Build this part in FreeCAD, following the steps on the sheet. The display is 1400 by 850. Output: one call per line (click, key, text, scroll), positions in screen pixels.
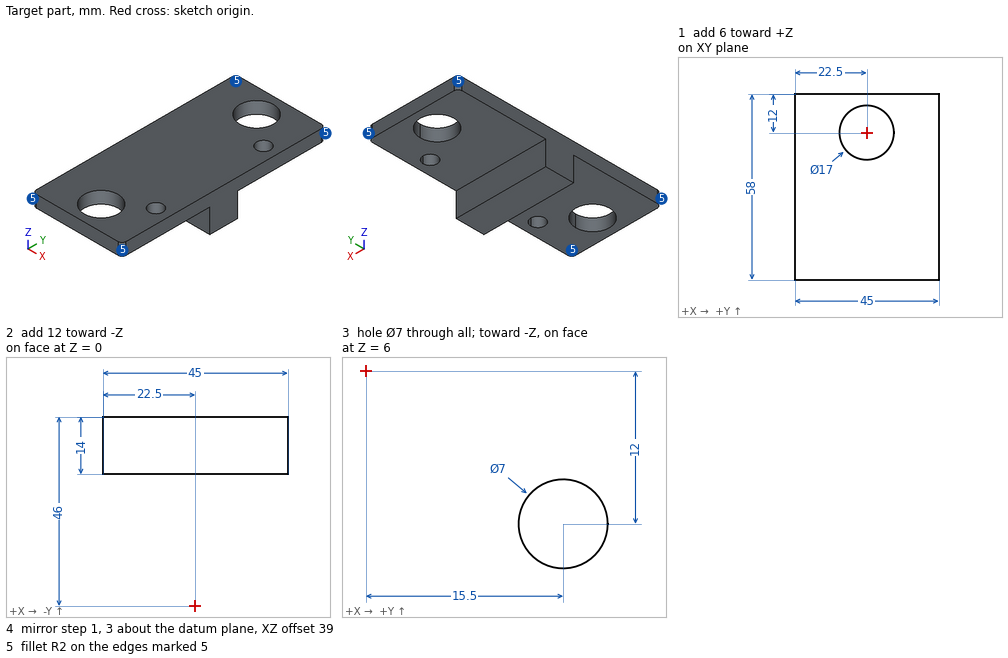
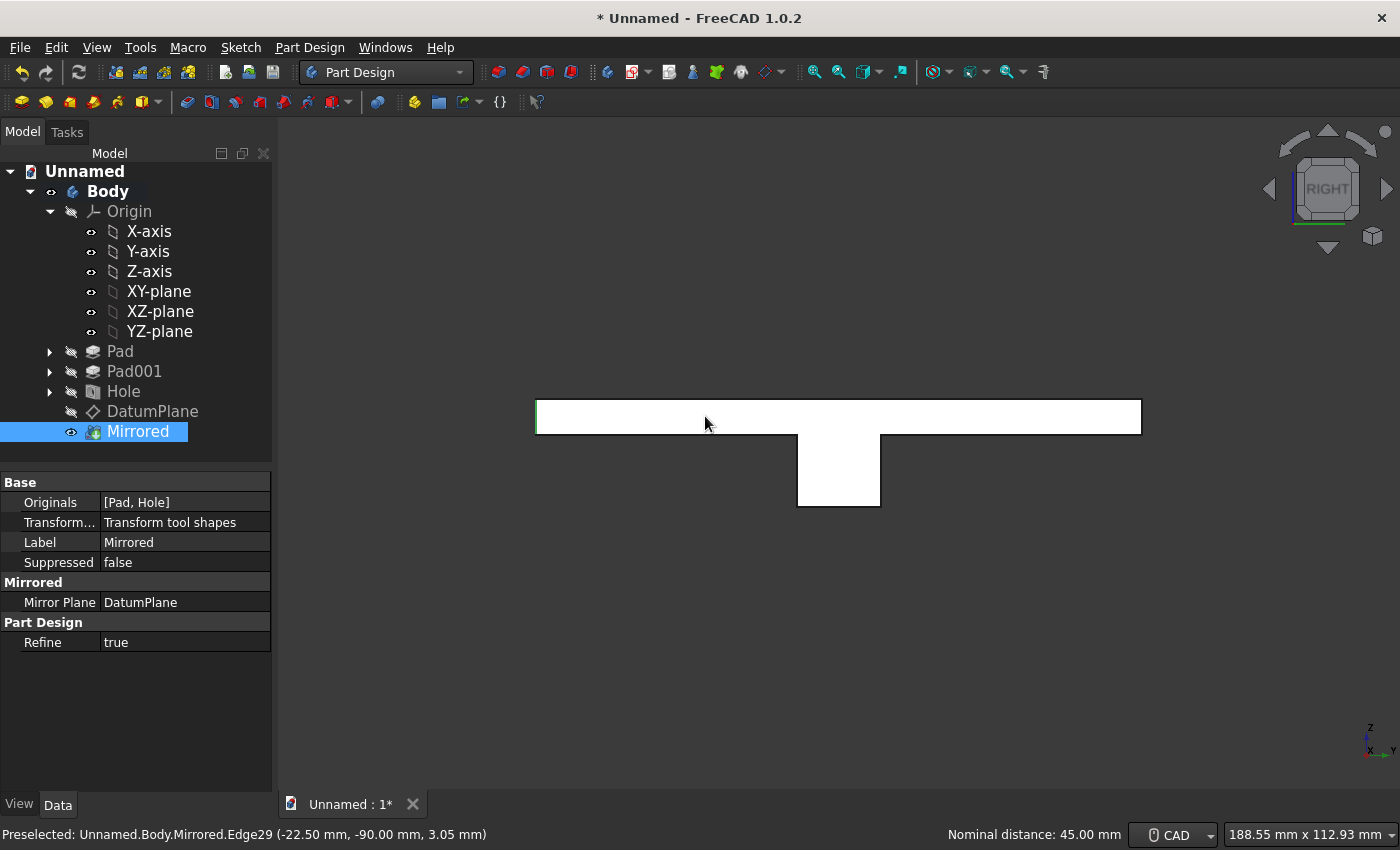
click(1142, 416, ctrl)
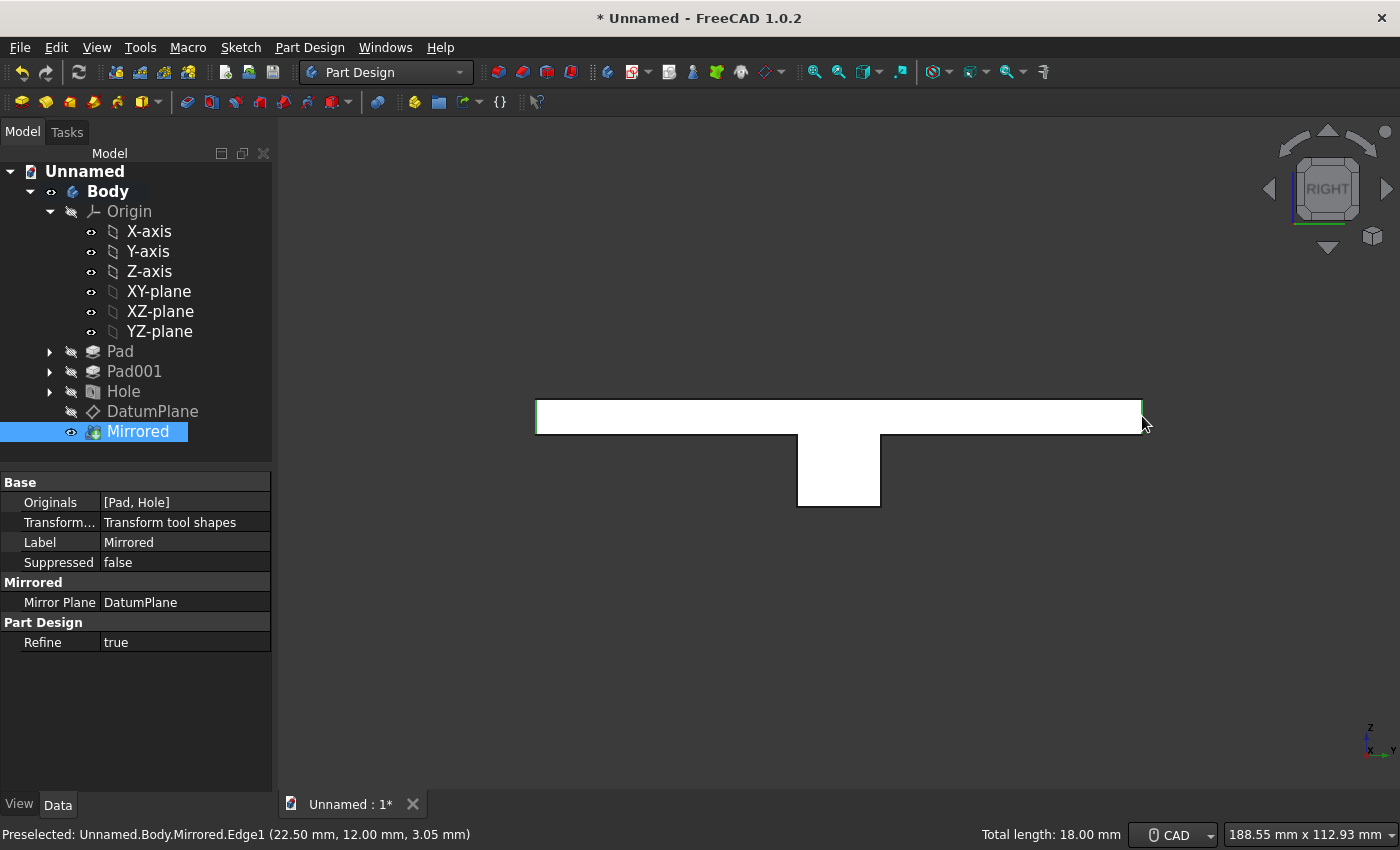
key(5)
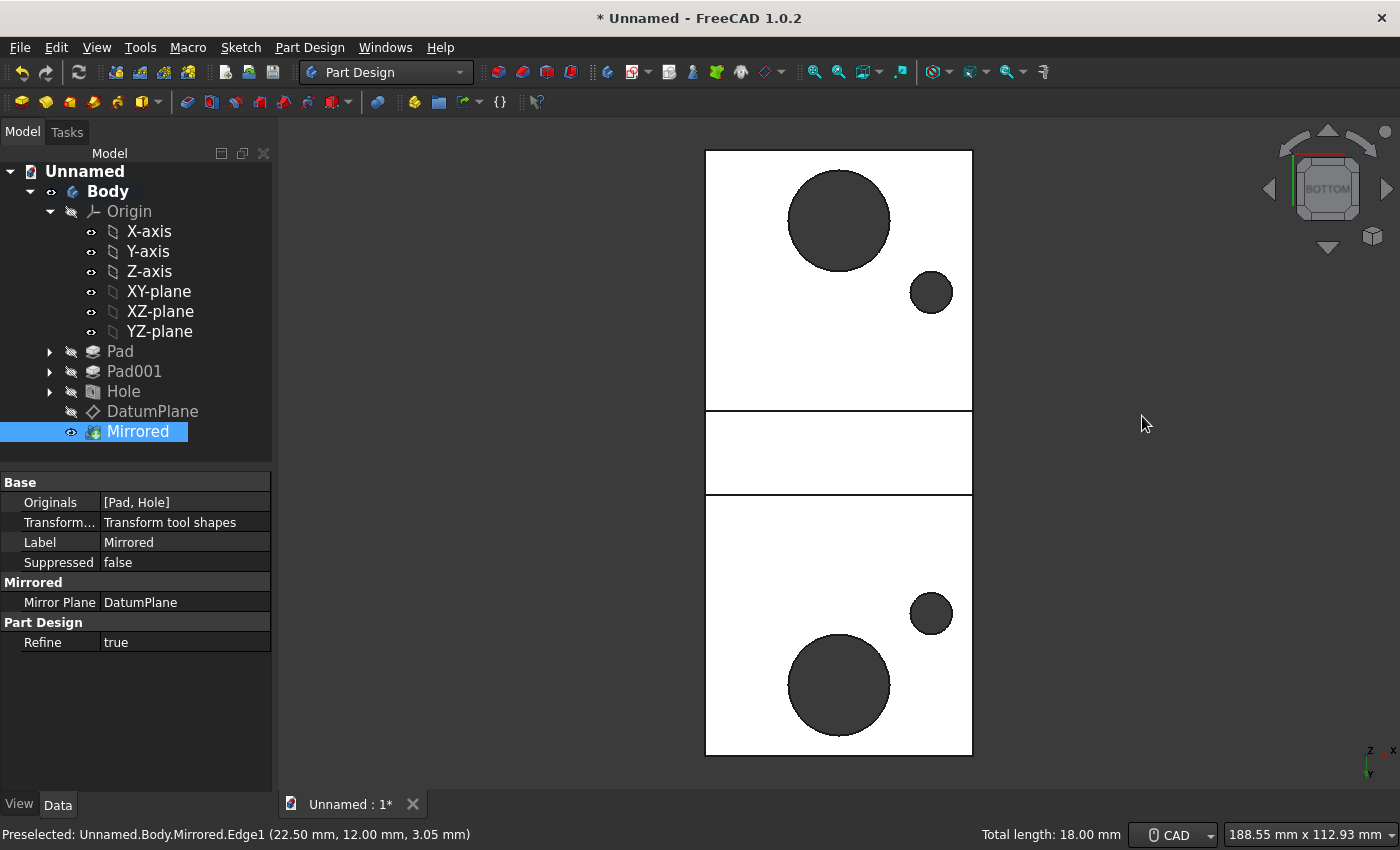
key(4)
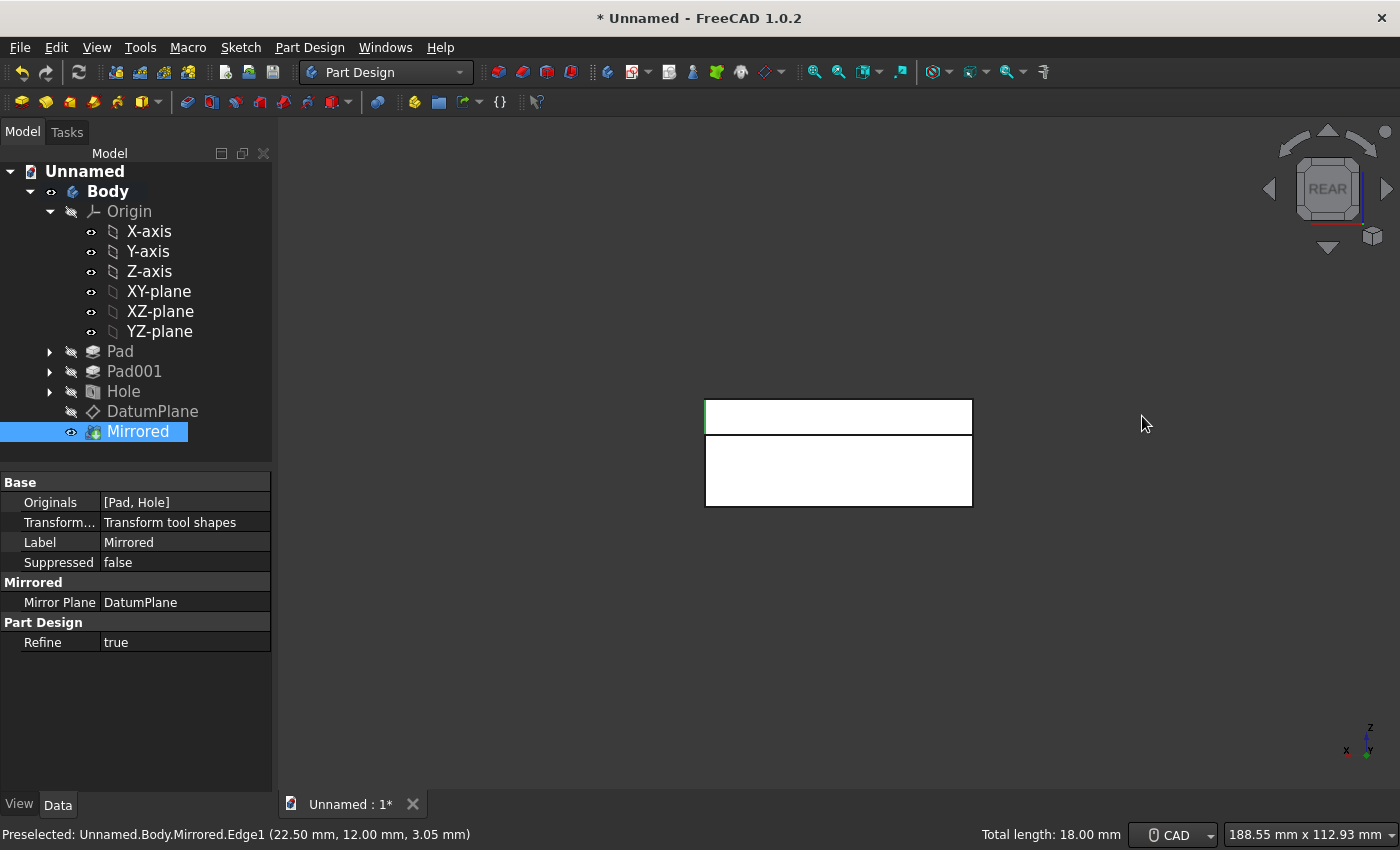
click(816, 72)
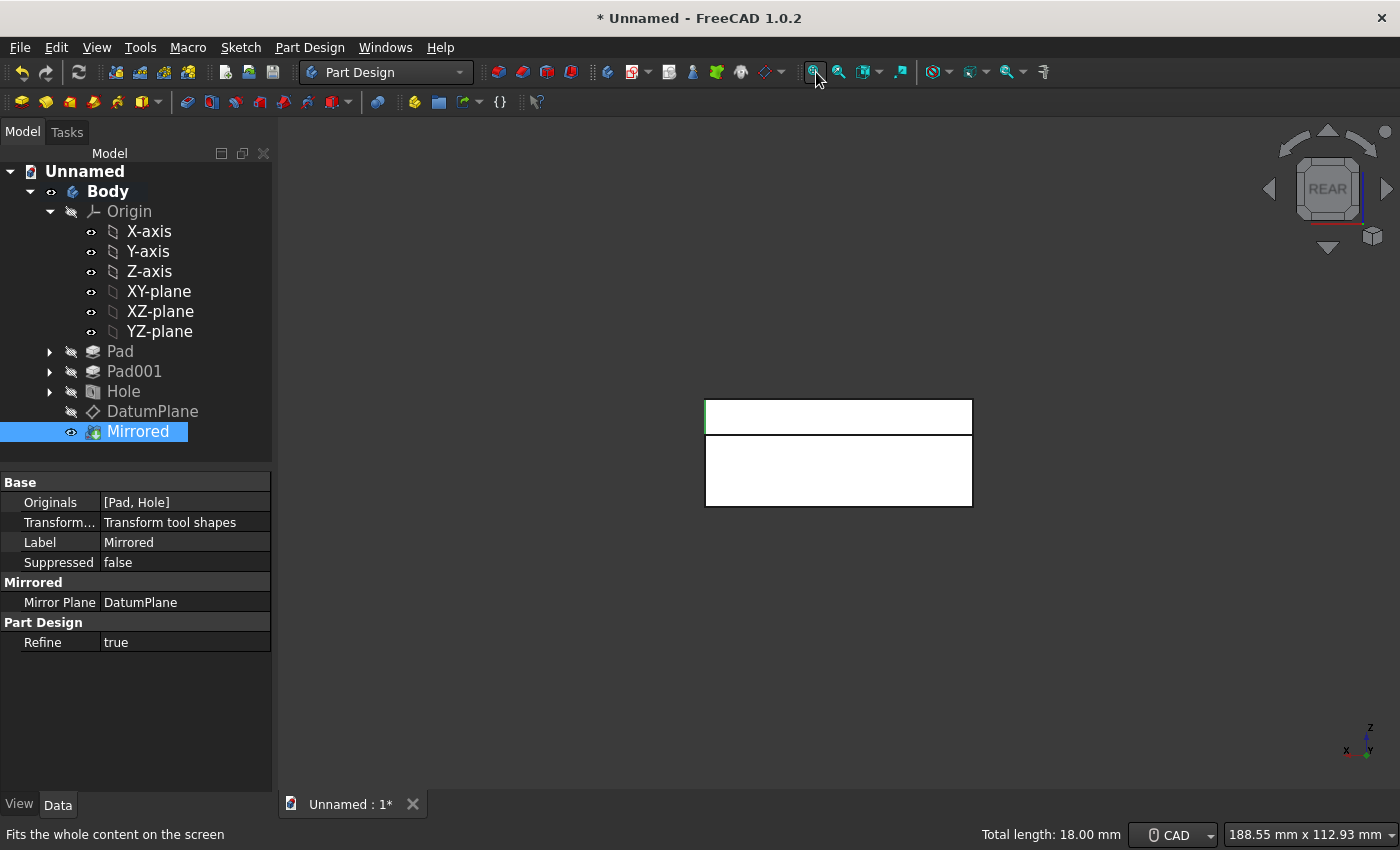
click(973, 416, ctrl)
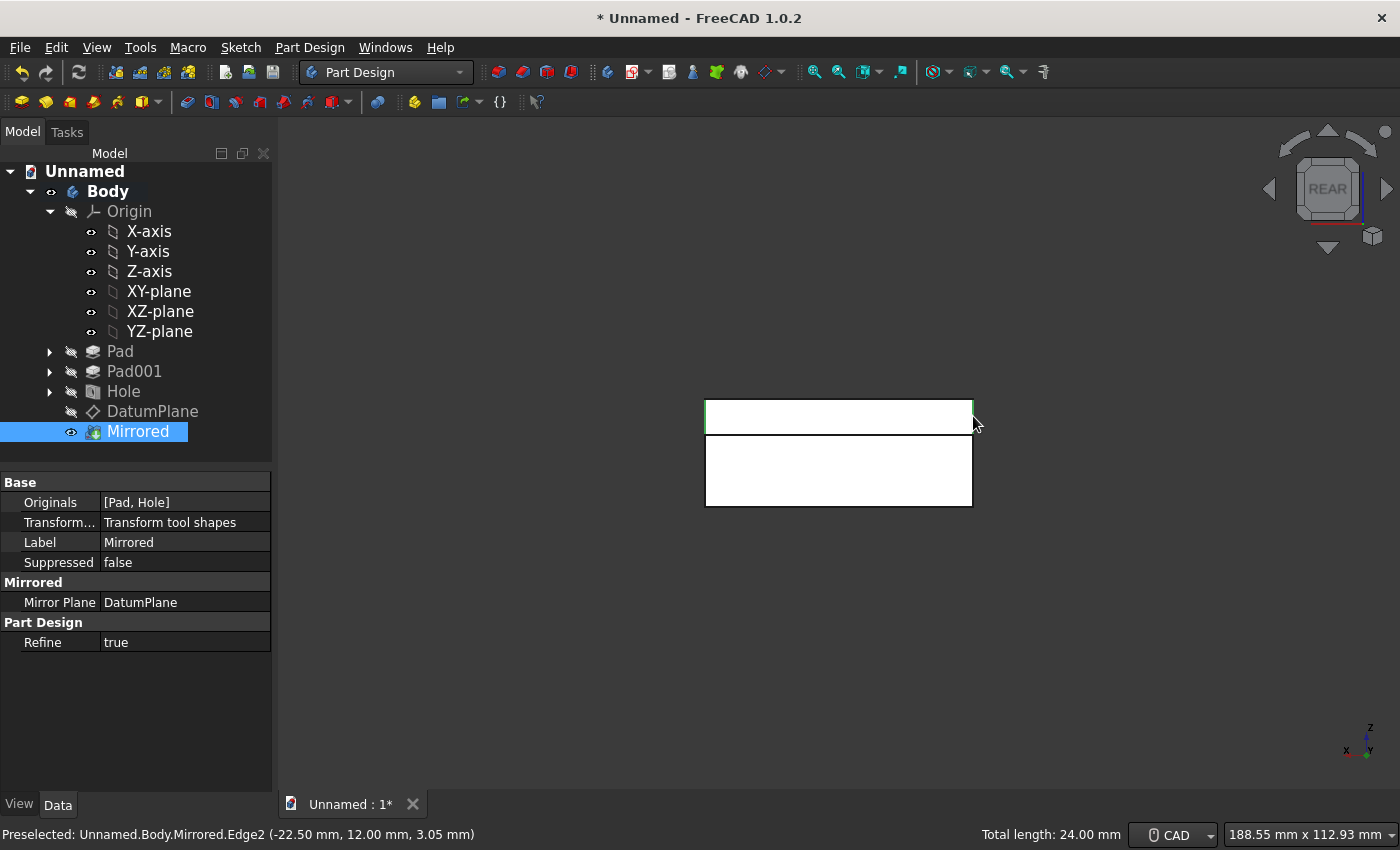
click(500, 72)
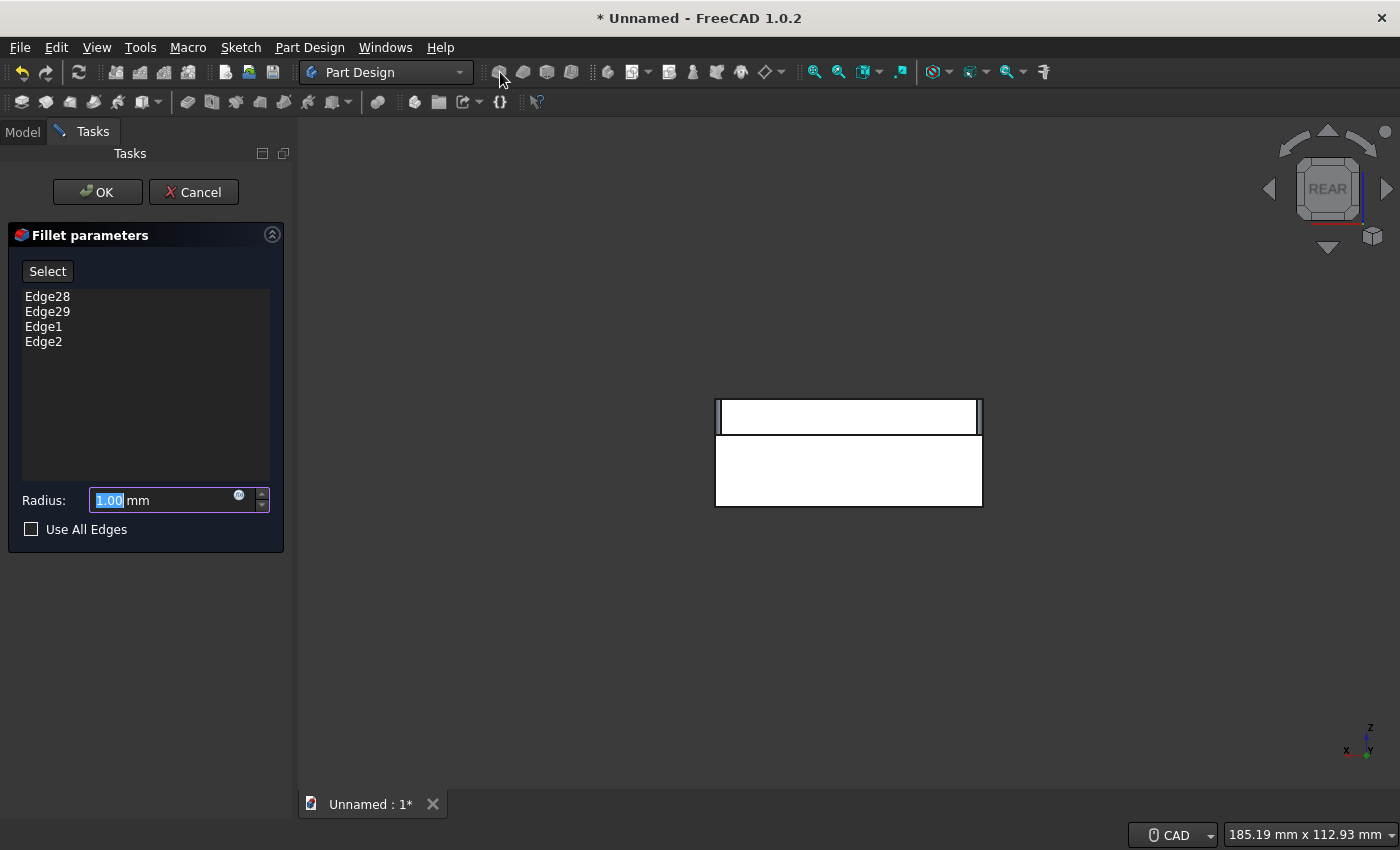
text(2)
key(Tab)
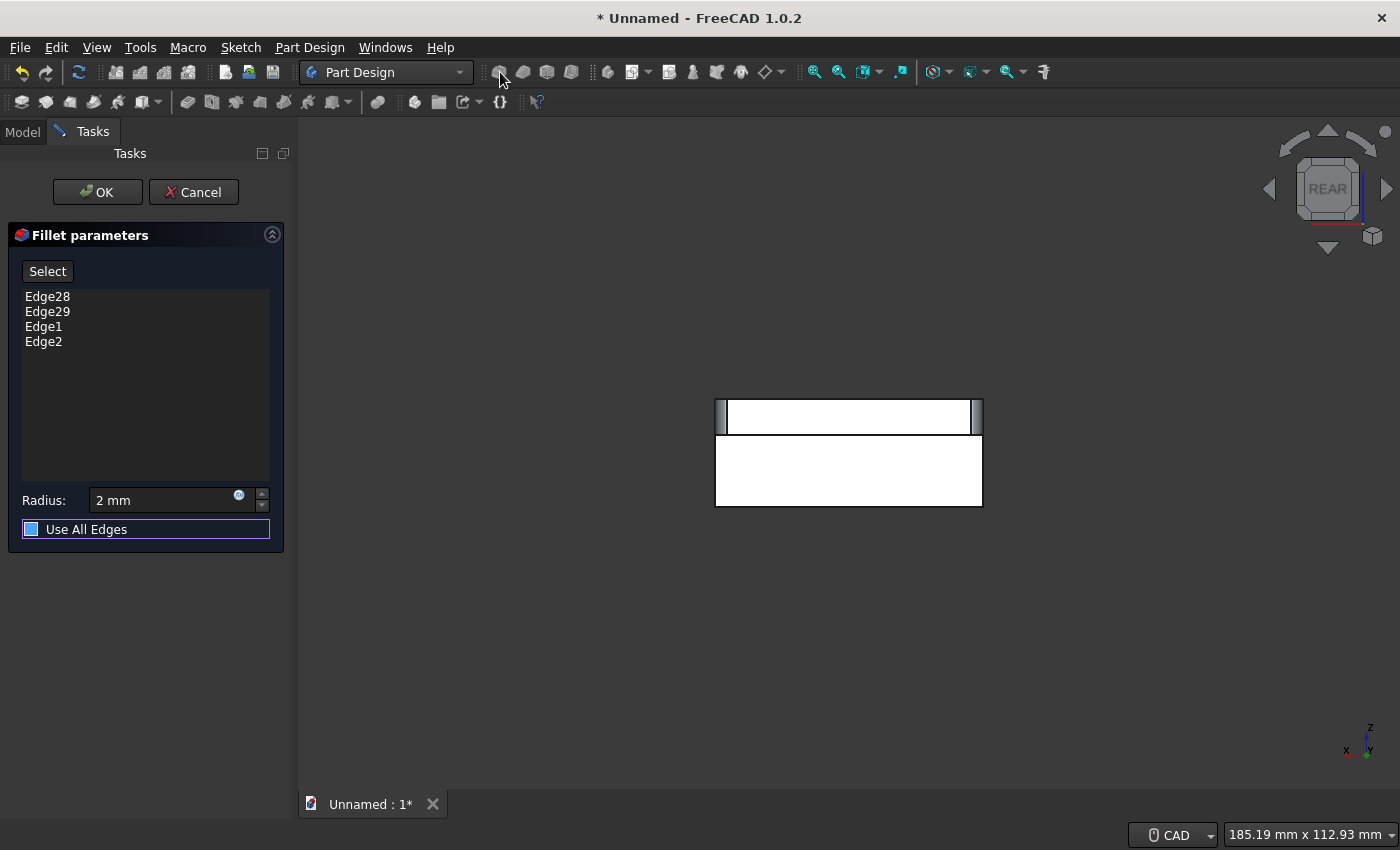
click(98, 192)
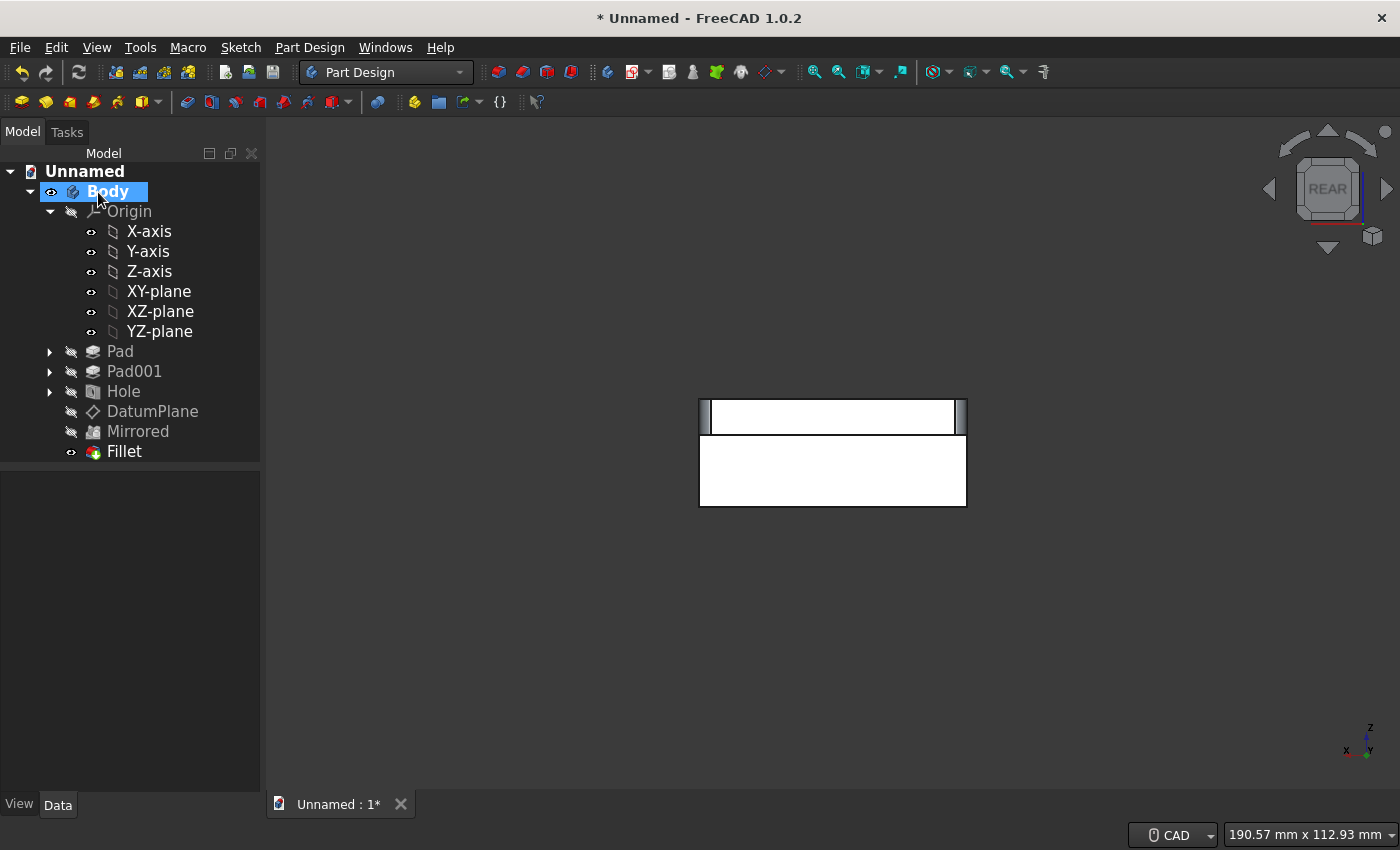
key(0)